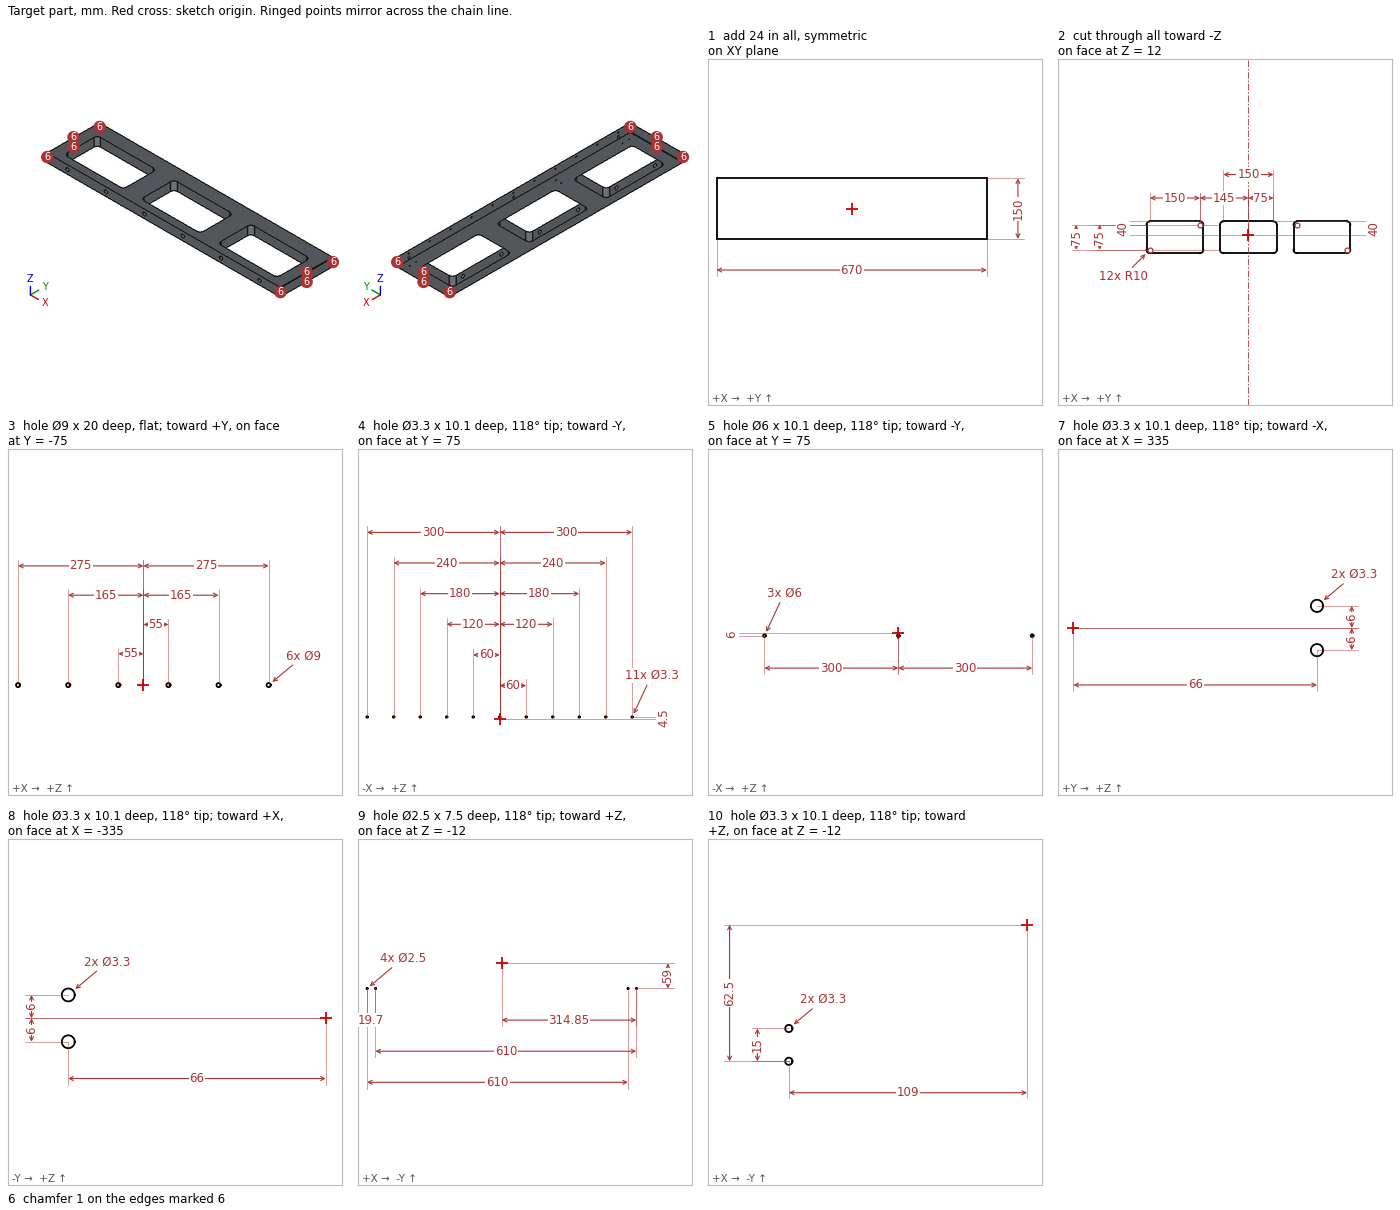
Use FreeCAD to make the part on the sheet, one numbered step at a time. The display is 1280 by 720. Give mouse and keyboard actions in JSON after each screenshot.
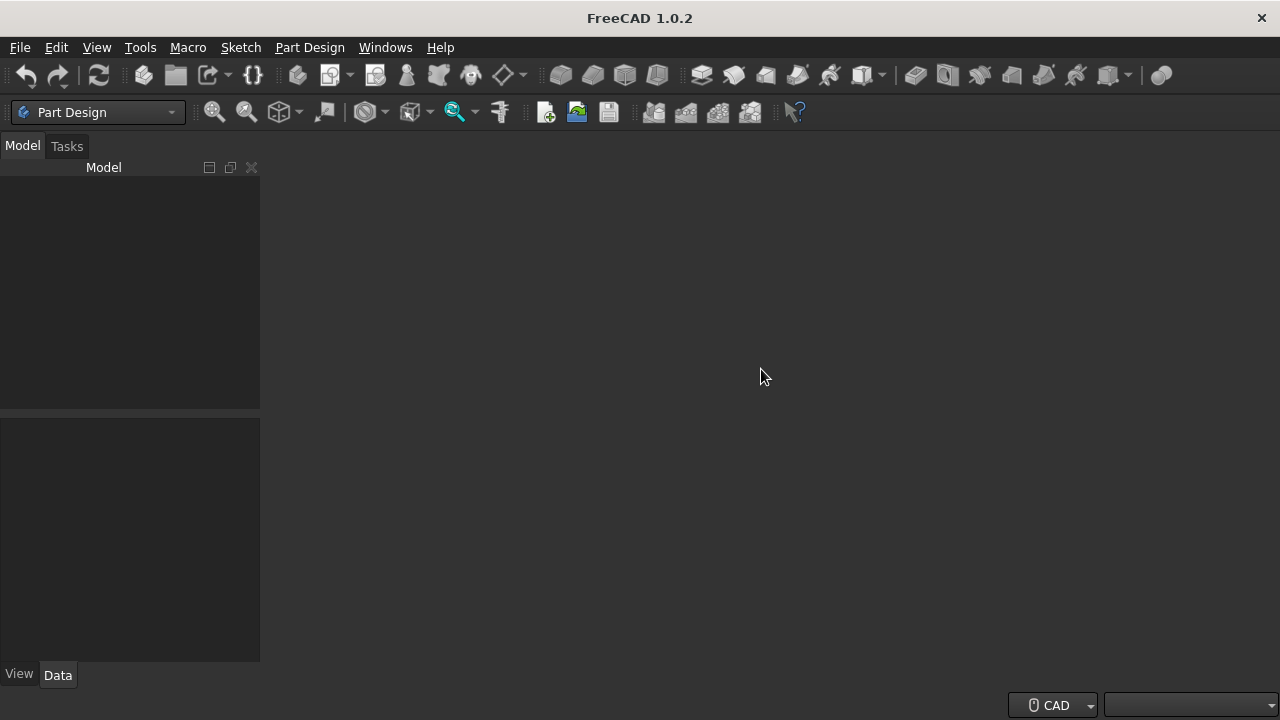
{"action": "left_click", "coordinate": [546, 112]}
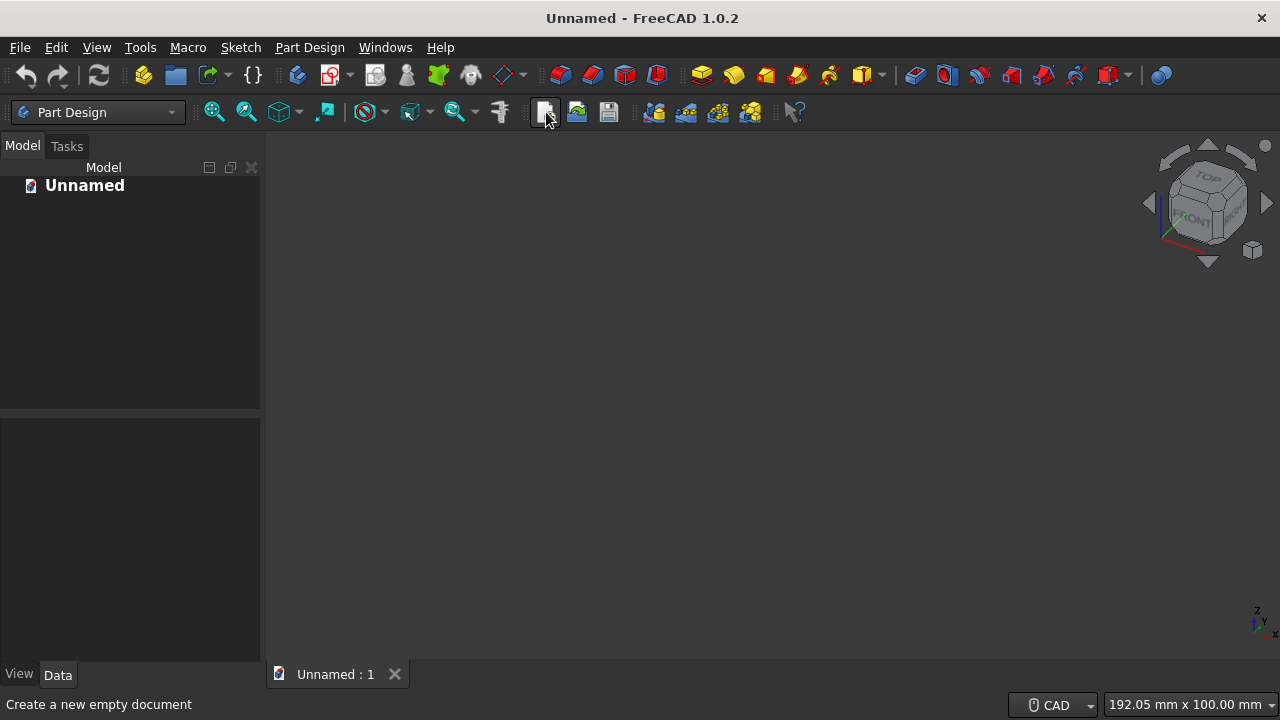
{"action": "left_click", "coordinate": [330, 76]}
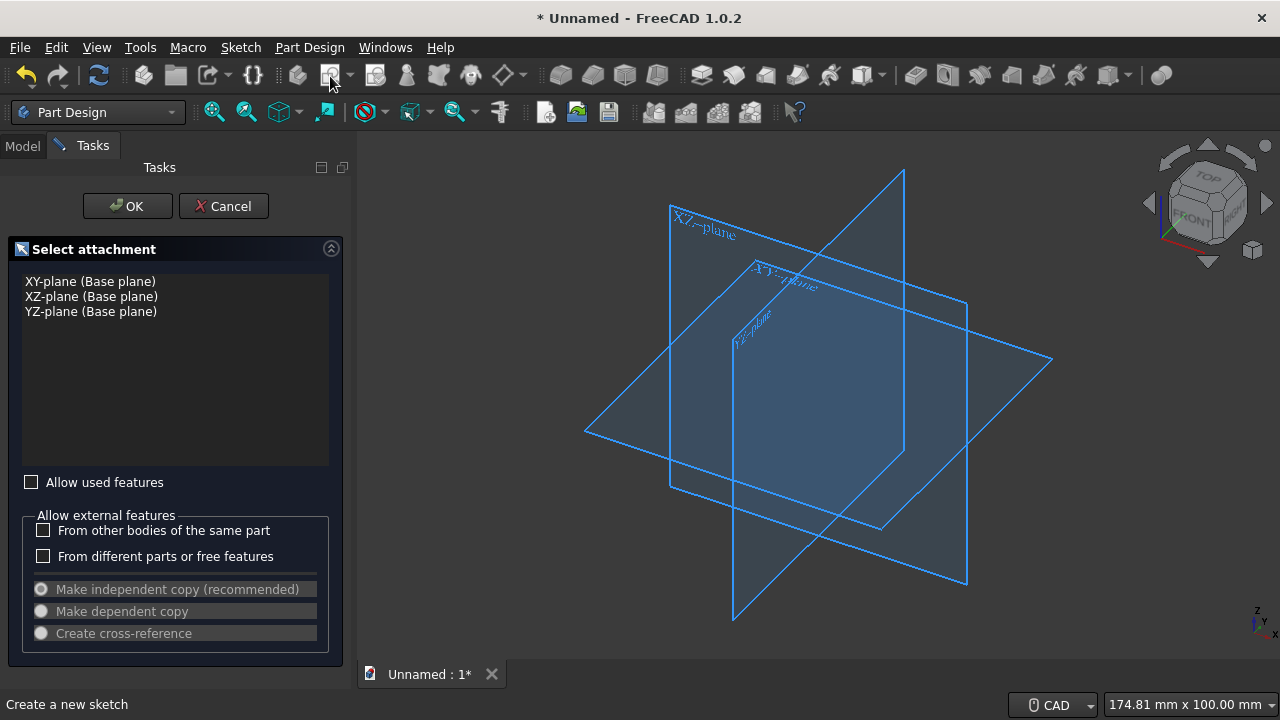
{"action": "left_click", "coordinate": [82, 282]}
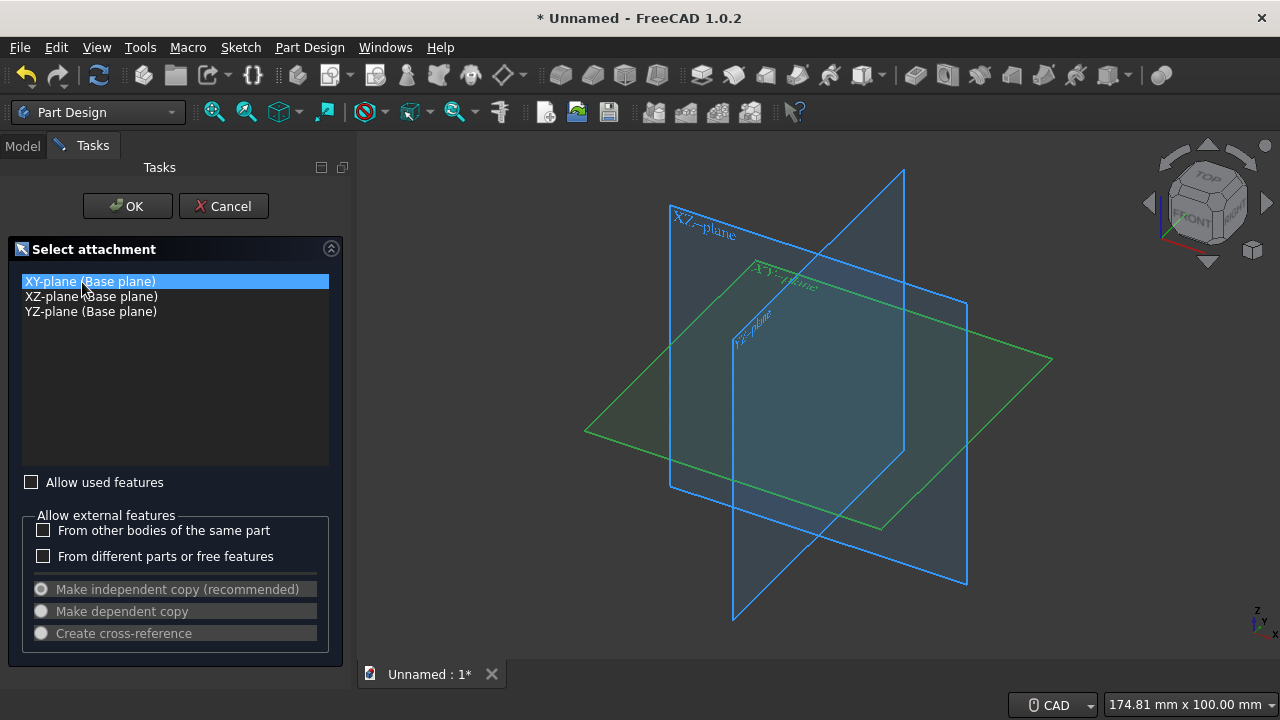
{"action": "left_click", "coordinate": [128, 206]}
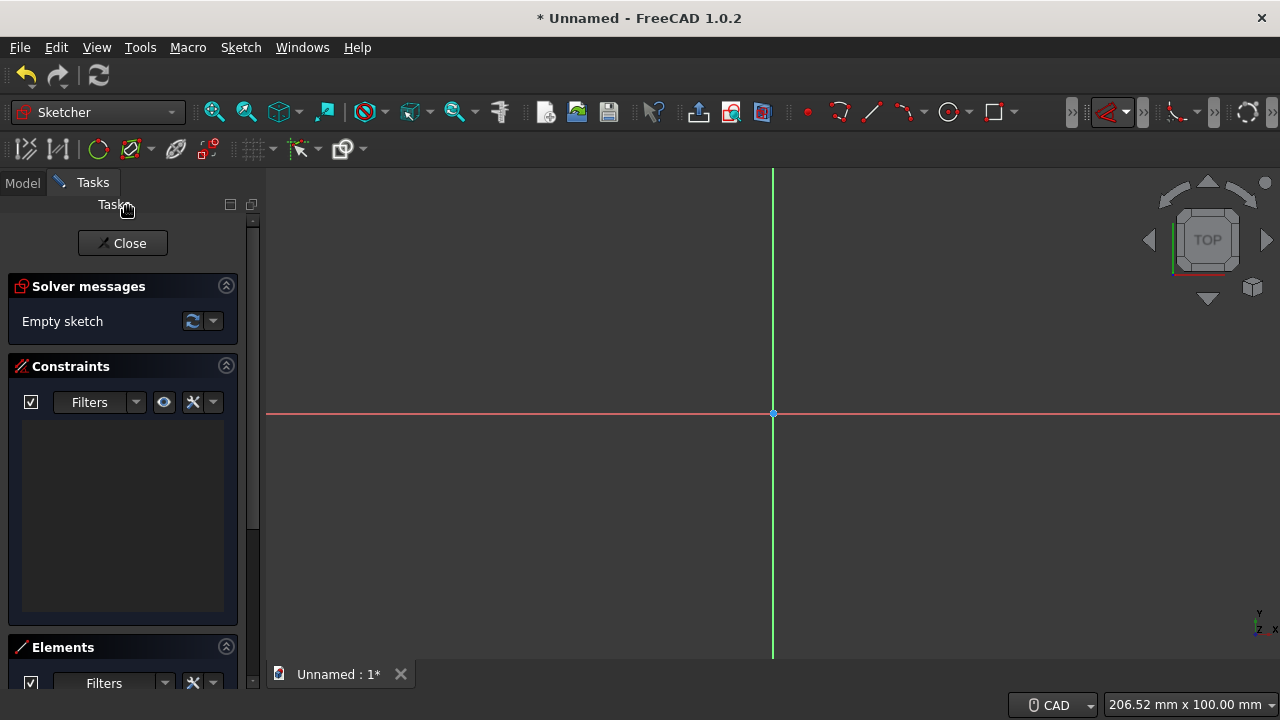
{"action": "scroll", "coordinate": [691, 414], "scroll_direction": "down", "scroll_amount": 9}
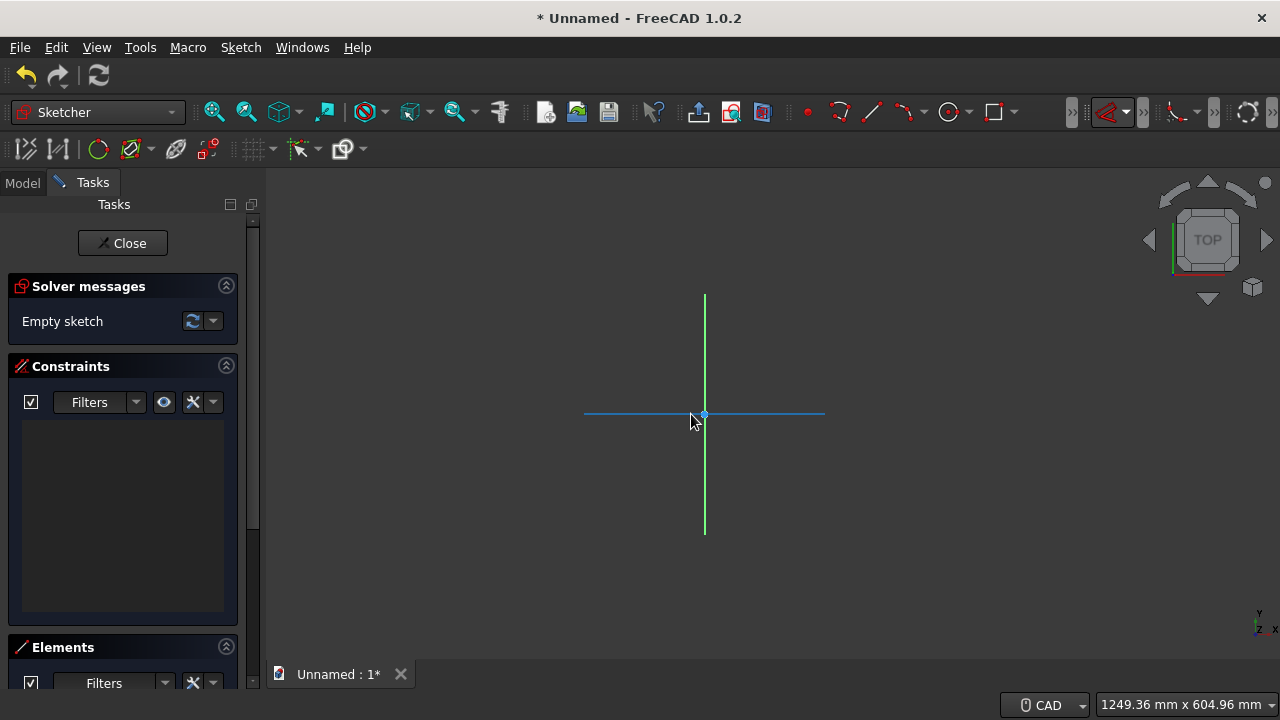
{"action": "key", "text": "g v"}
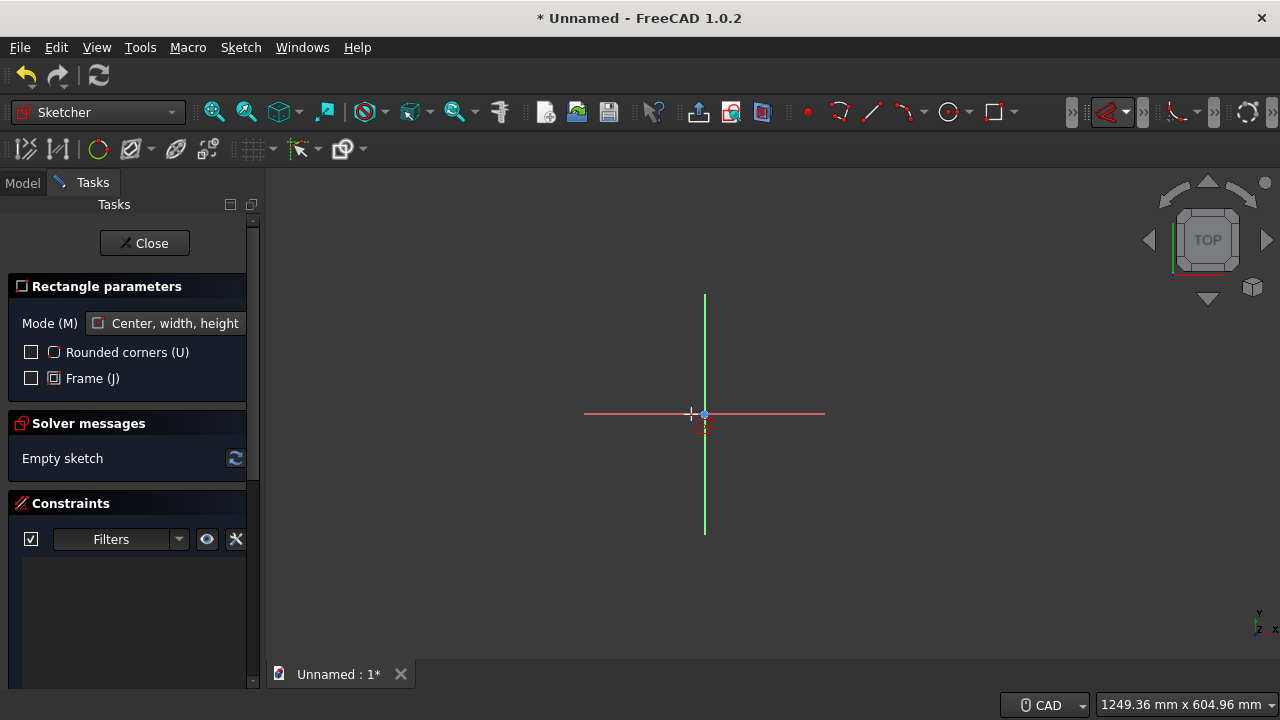
{"action": "left_click", "coordinate": [705, 414]}
{"action": "mouse_move", "coordinate": [977, 353]}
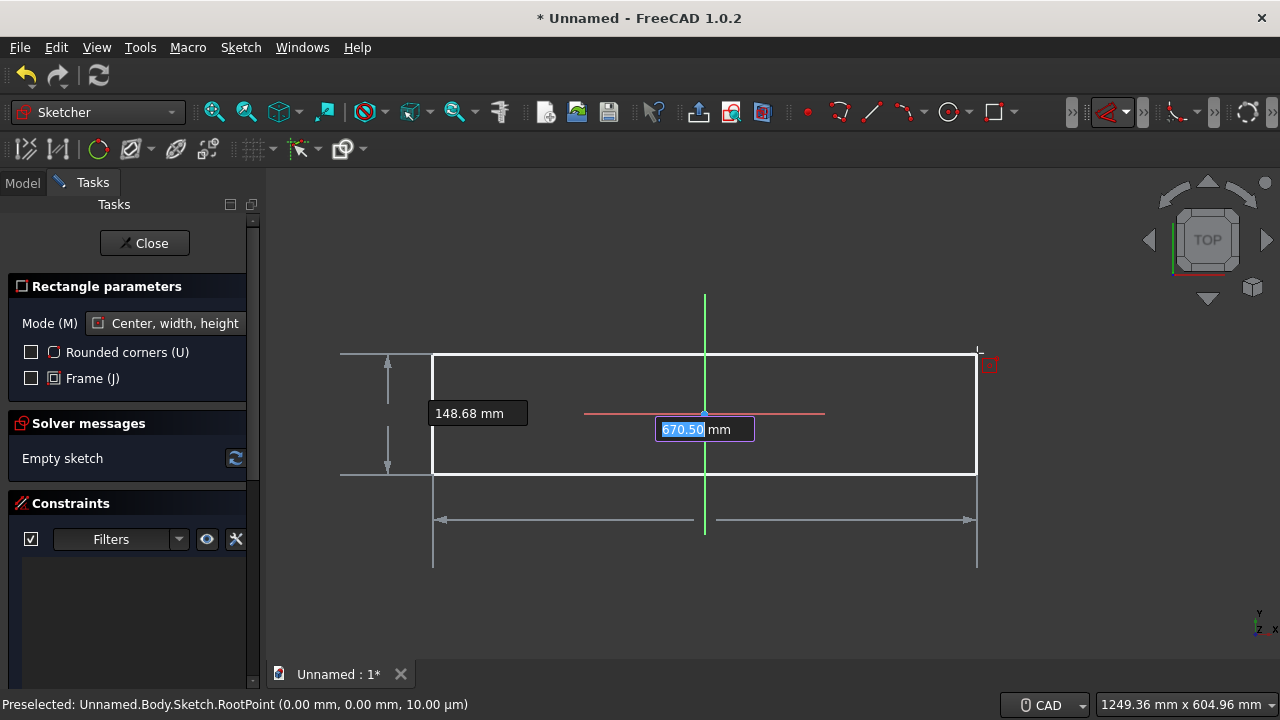
{"action": "type", "text": "670"}
{"action": "key", "text": "Tab"}
{"action": "type", "text": "150"}
{"action": "key", "text": "Return"}
{"action": "key", "text": "Escape"}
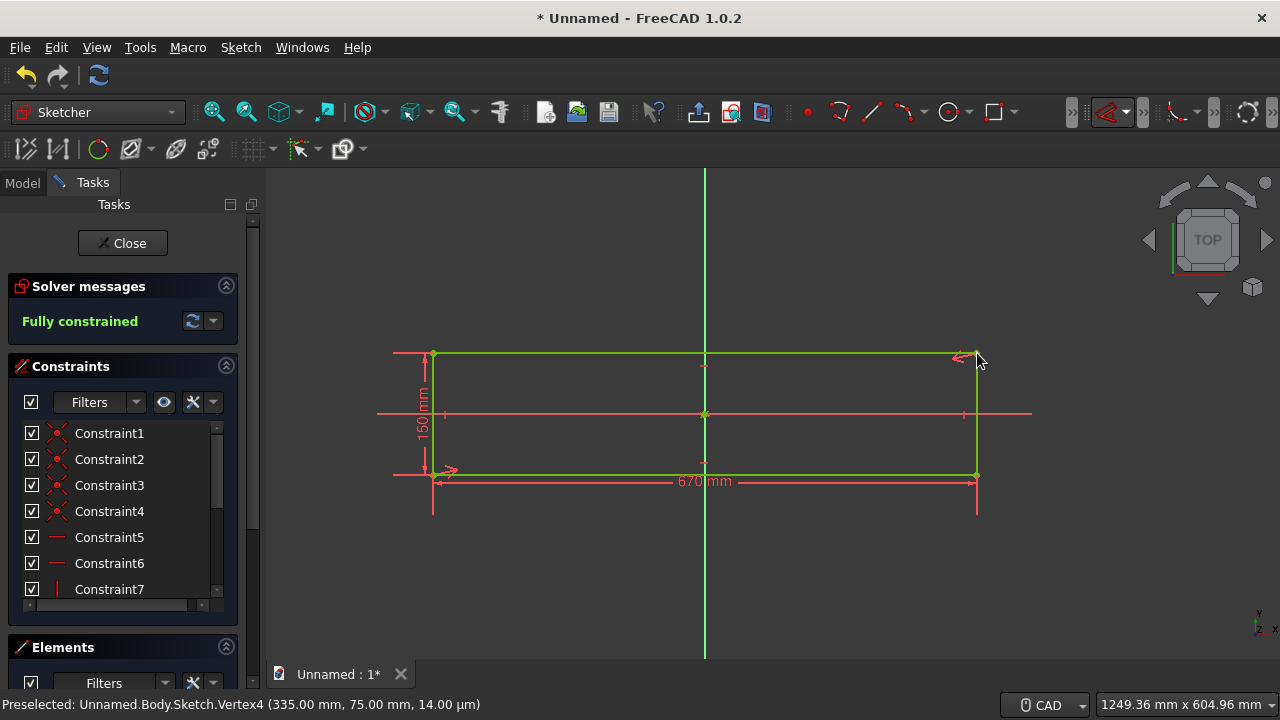
{"action": "left_click", "coordinate": [123, 243]}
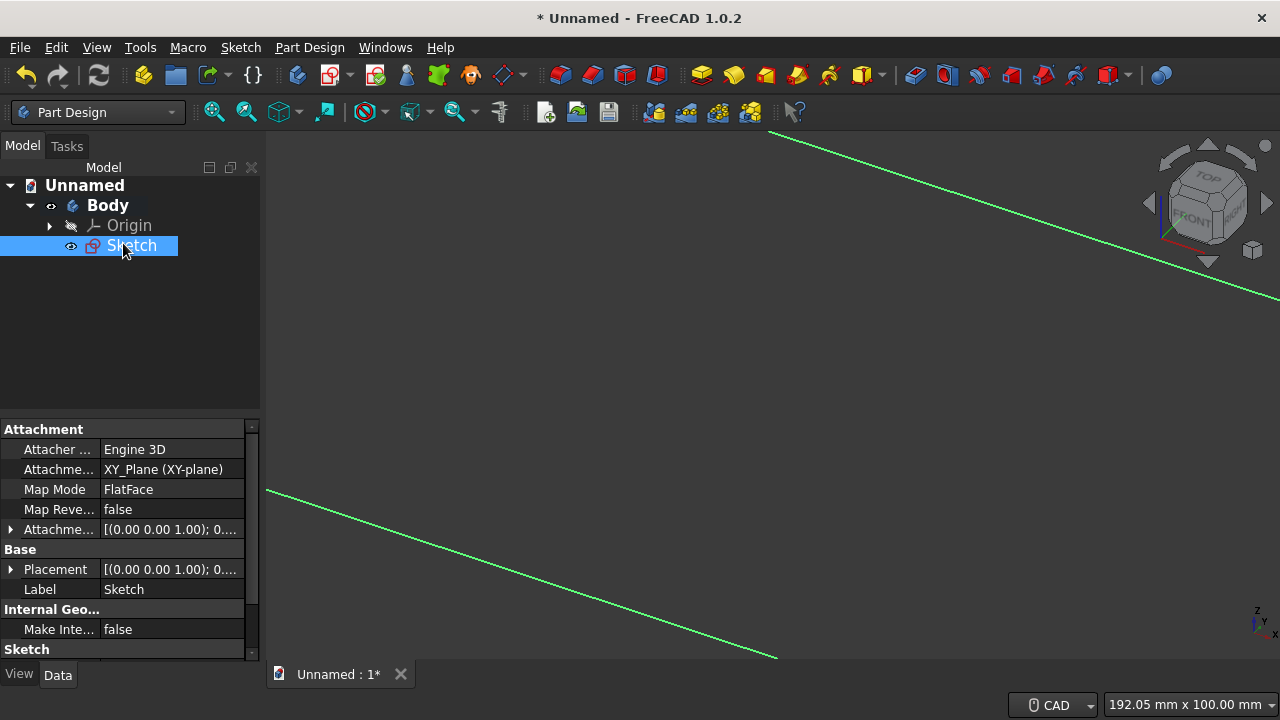
{"action": "left_click", "coordinate": [702, 76]}